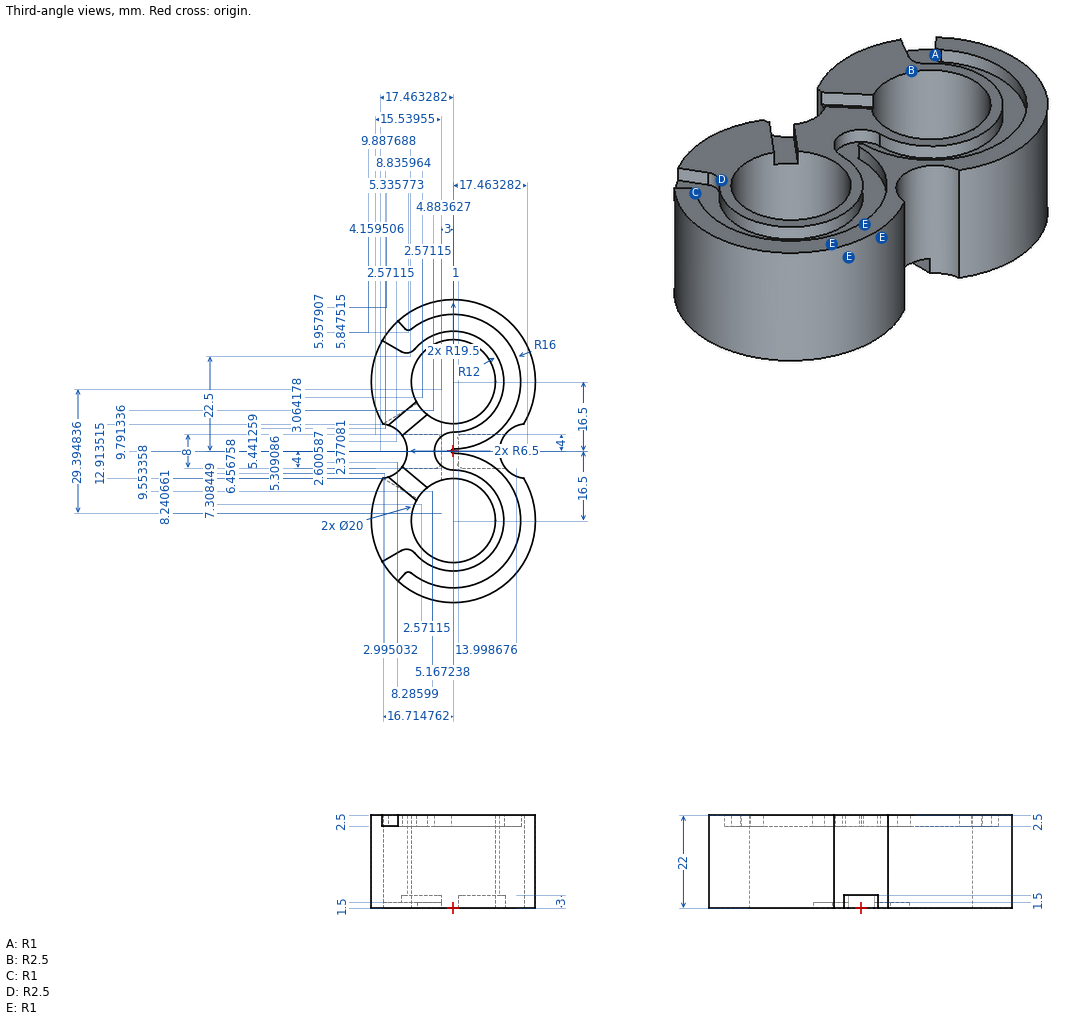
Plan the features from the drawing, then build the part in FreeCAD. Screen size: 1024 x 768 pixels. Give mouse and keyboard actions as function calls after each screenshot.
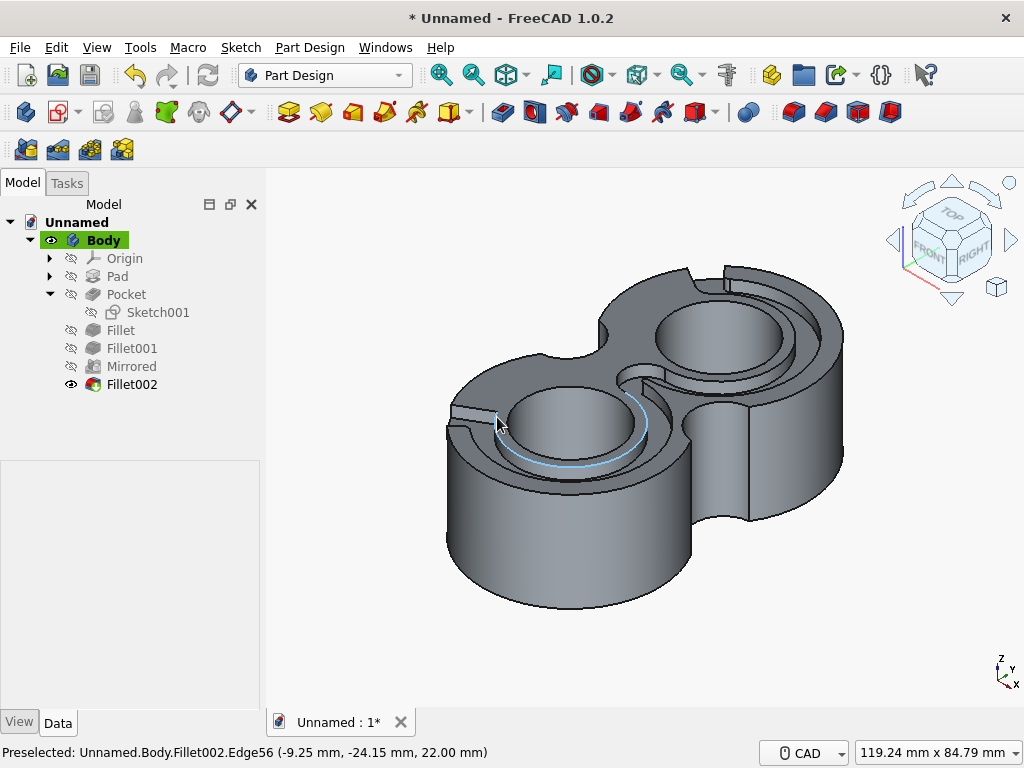
key(2)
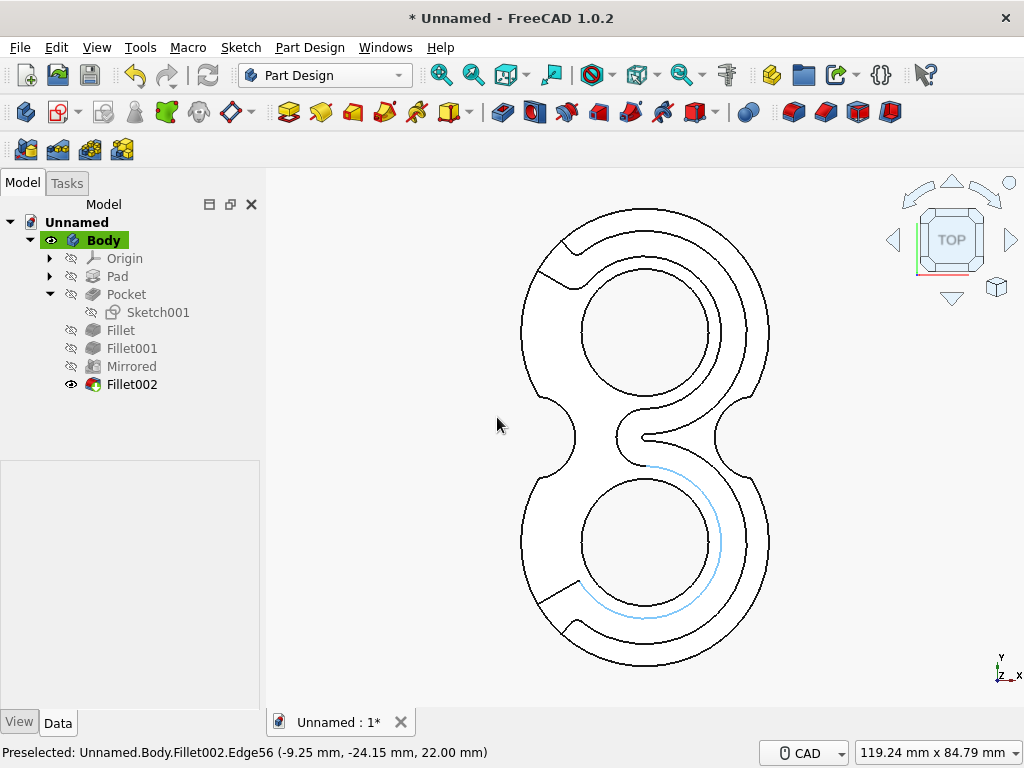
scroll(579, 580, up, 5)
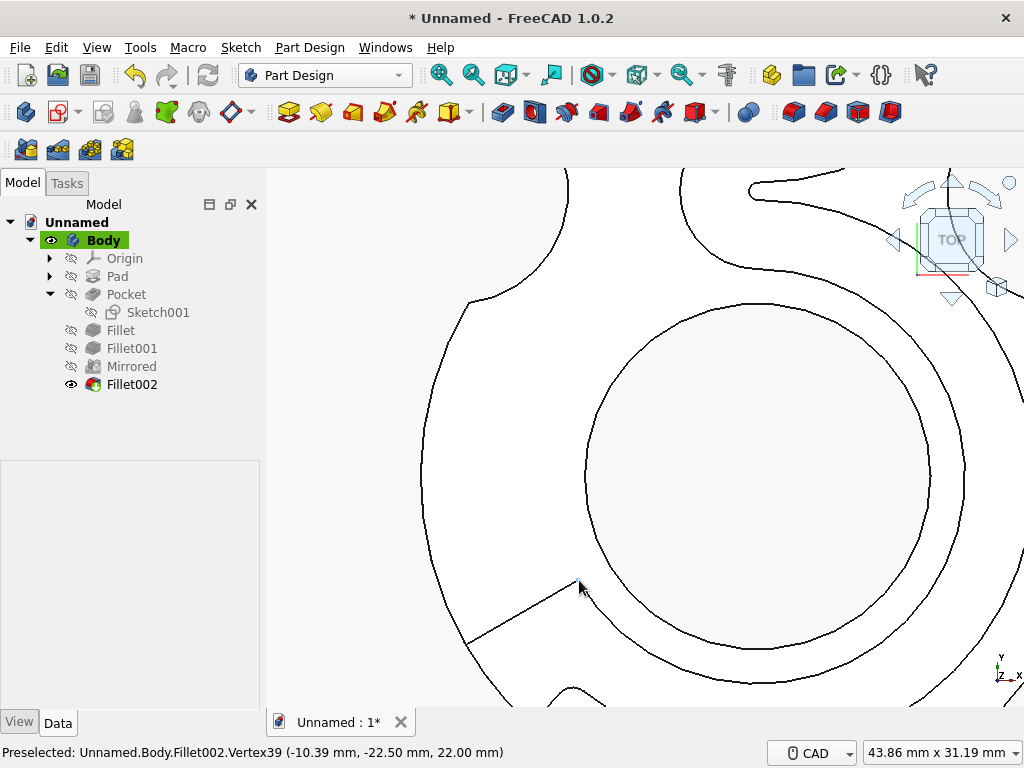
click(442, 76)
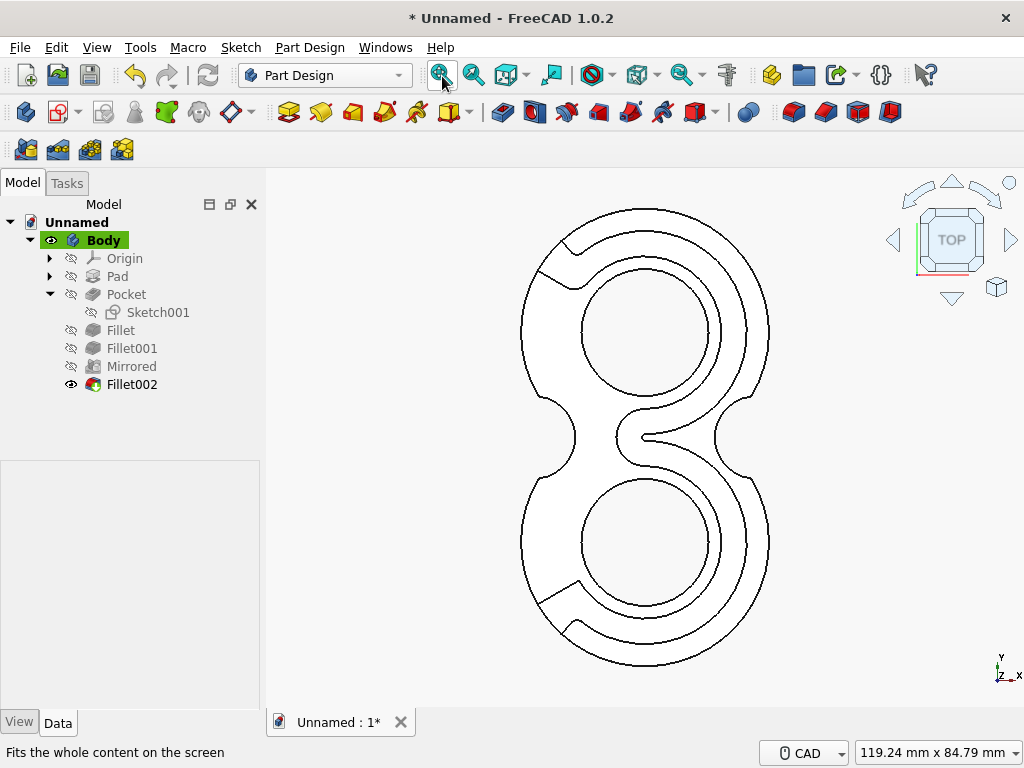
key(0)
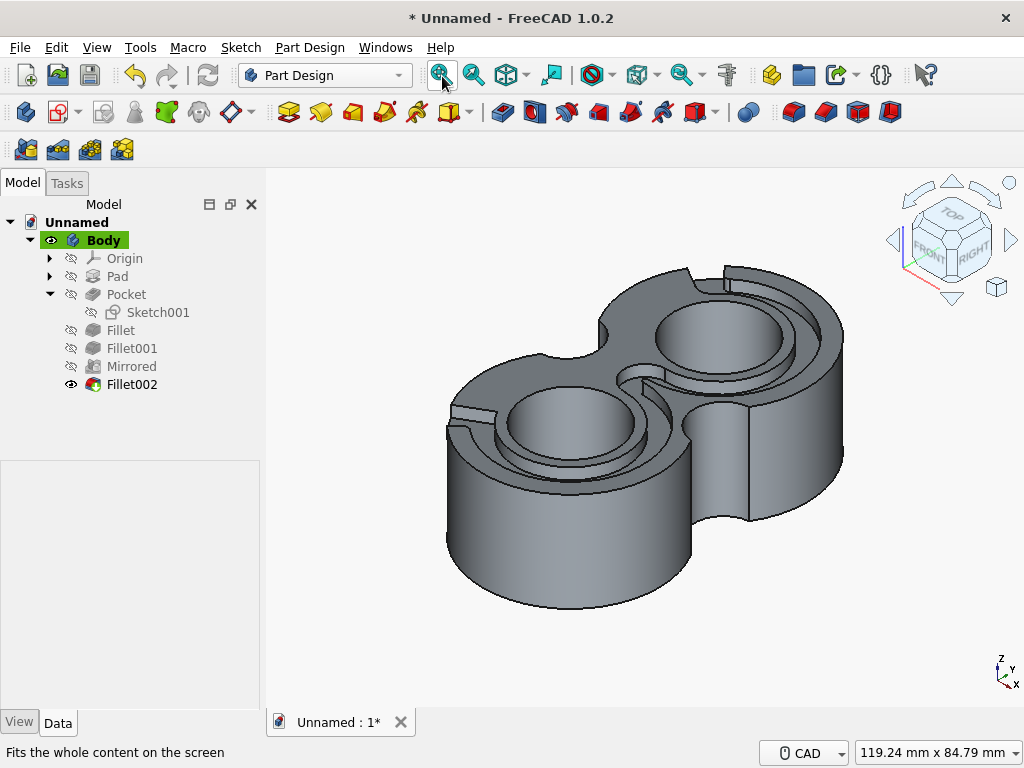
scroll(497, 417, up, 5)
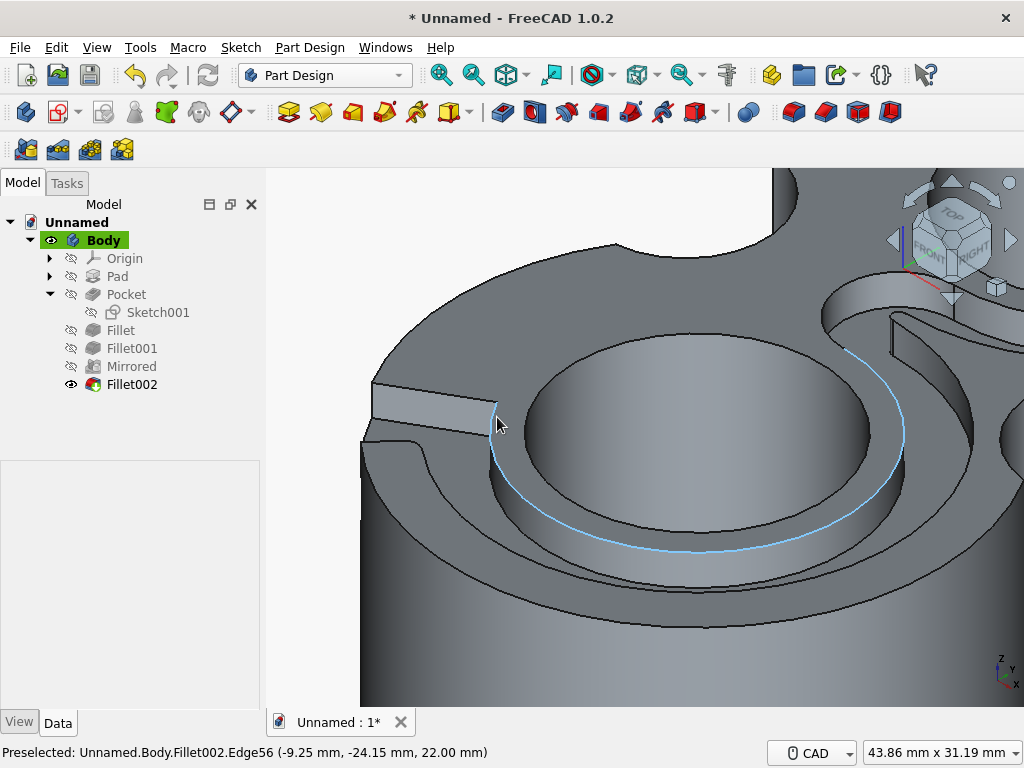
key(v)
key(f)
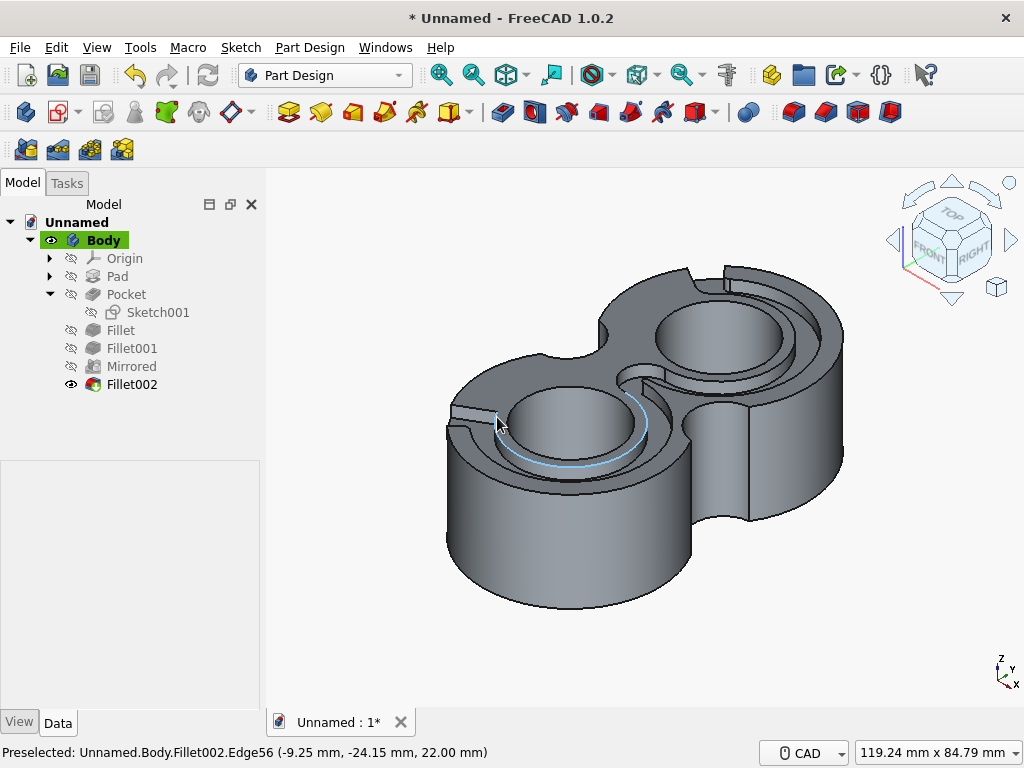
key(1)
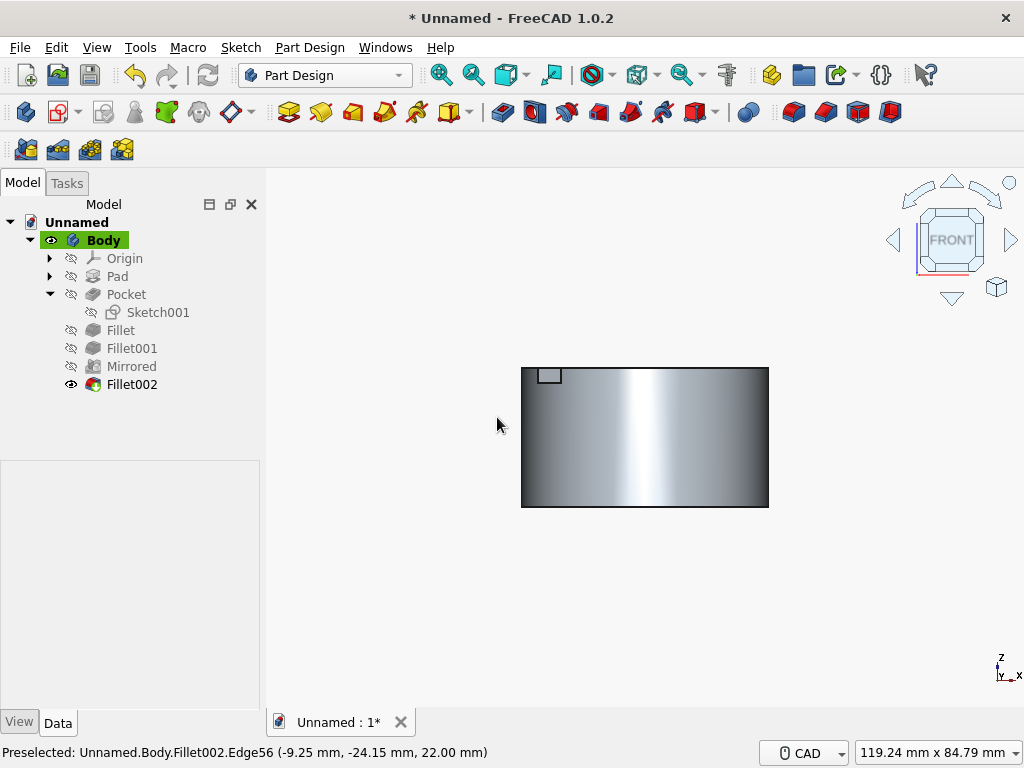
key(v)
key(f)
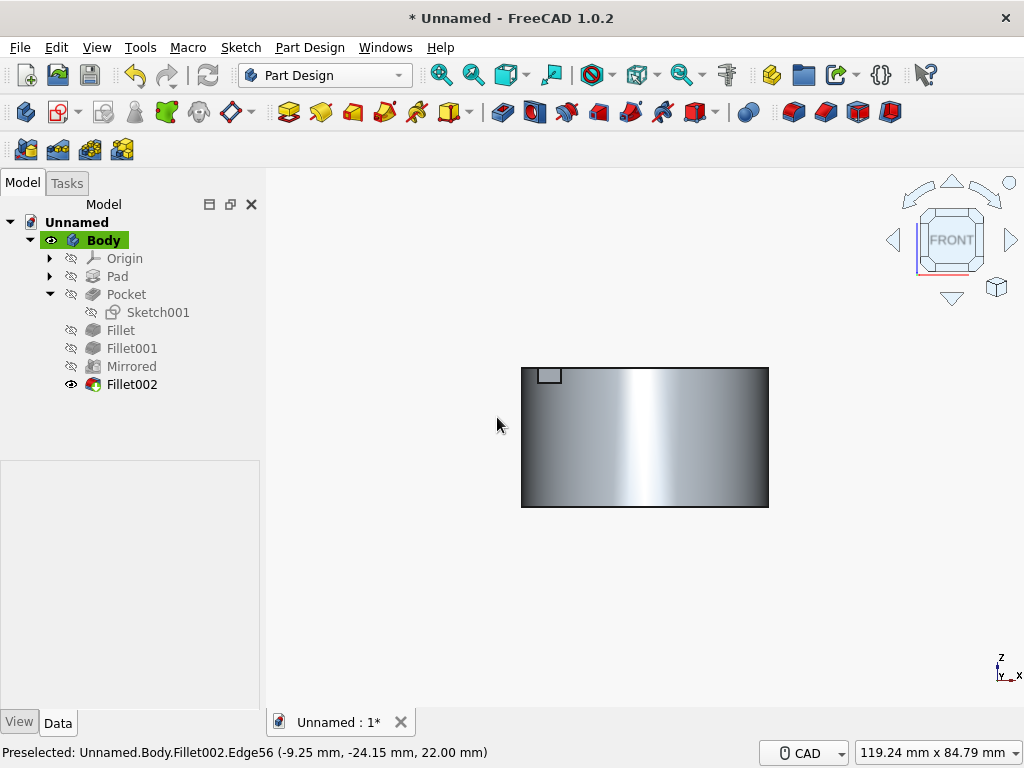
scroll(579, 375, up, 5)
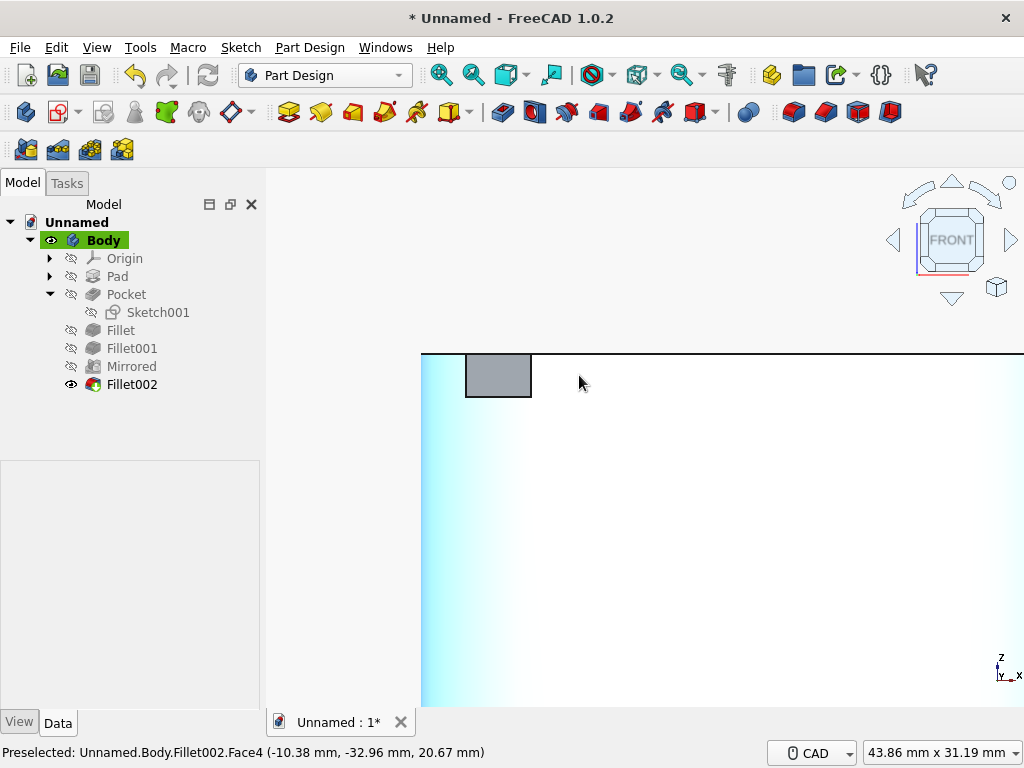
click(442, 76)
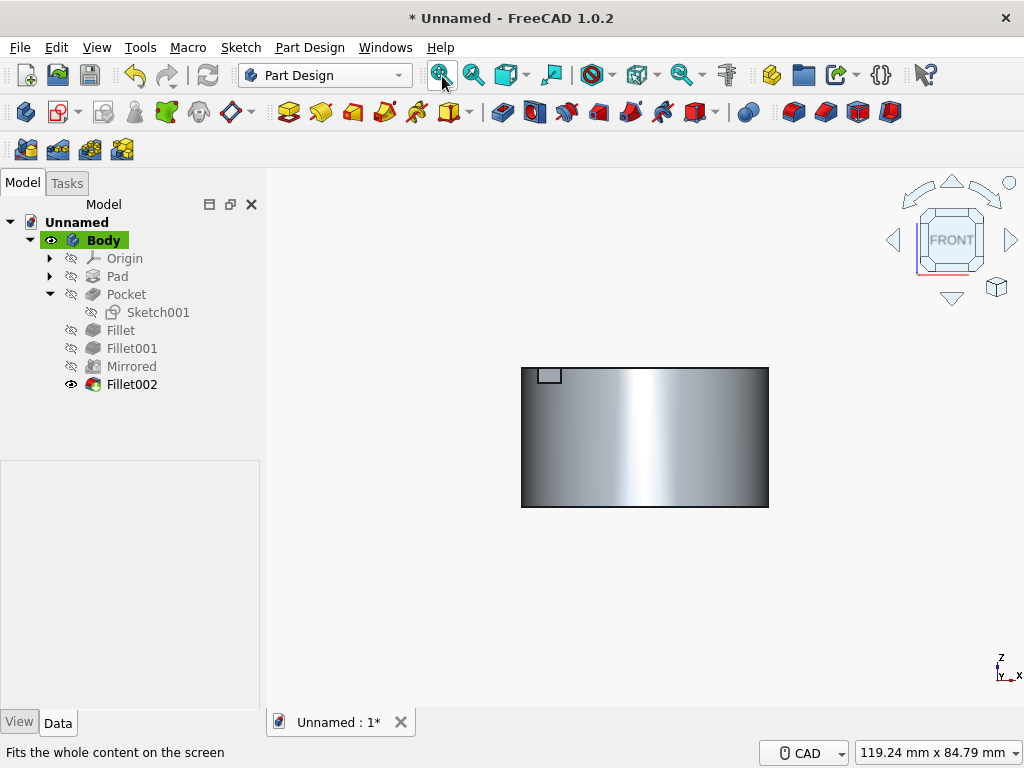
key(3)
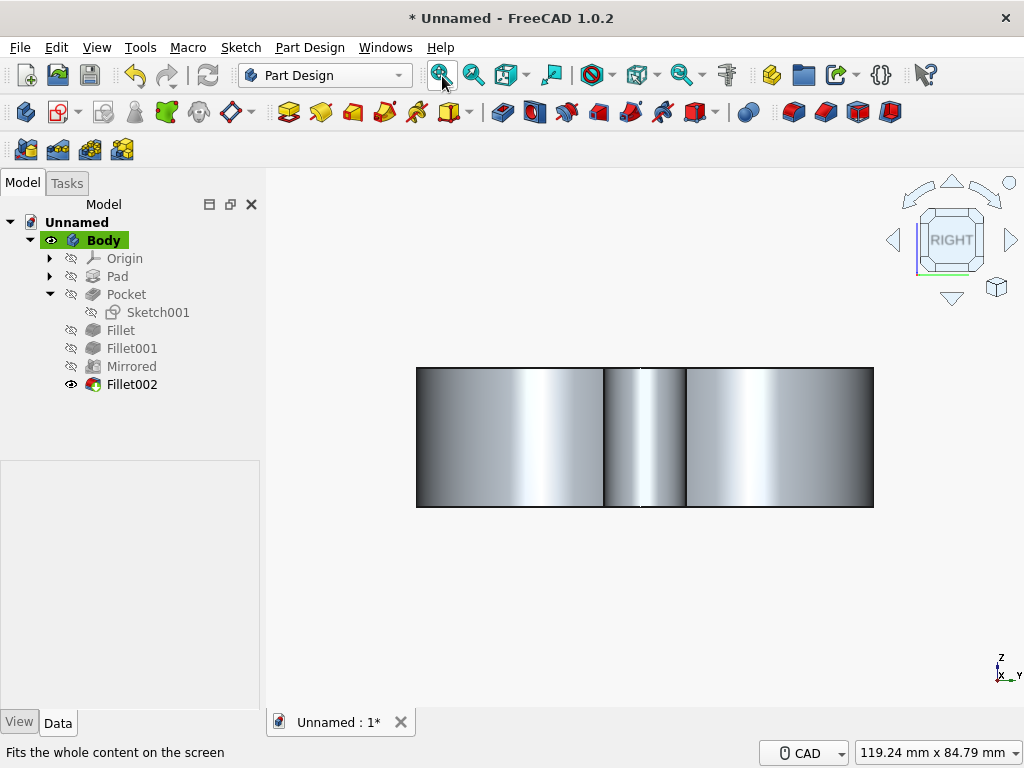
scroll(502, 375, up, 5)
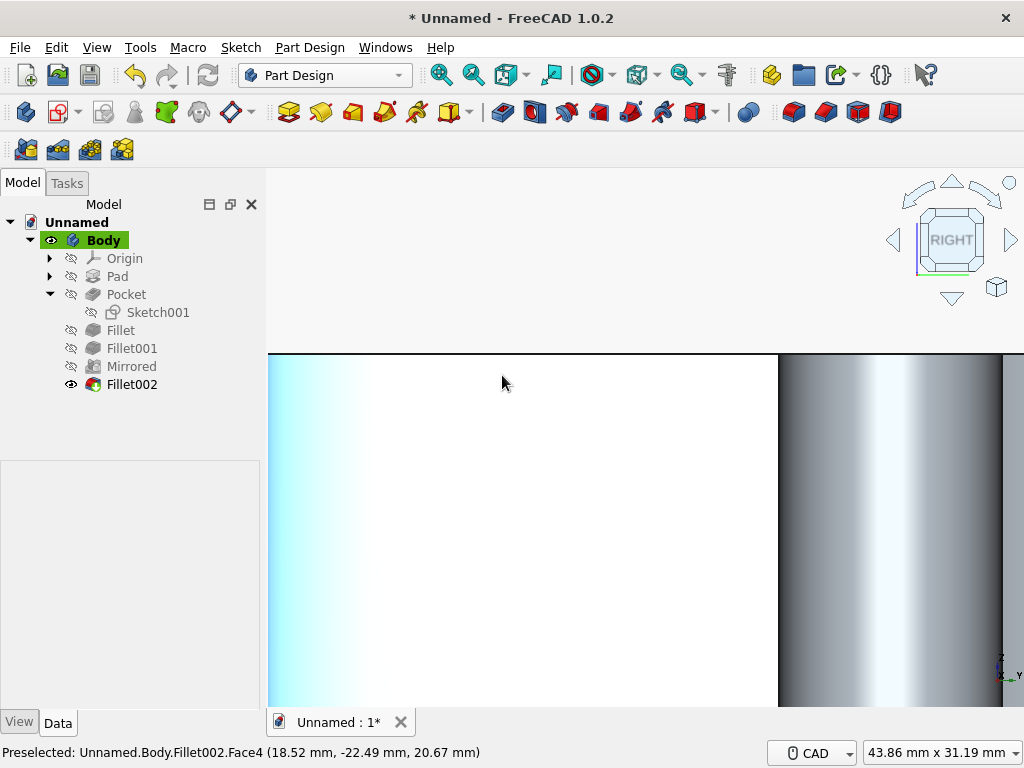
click(442, 76)